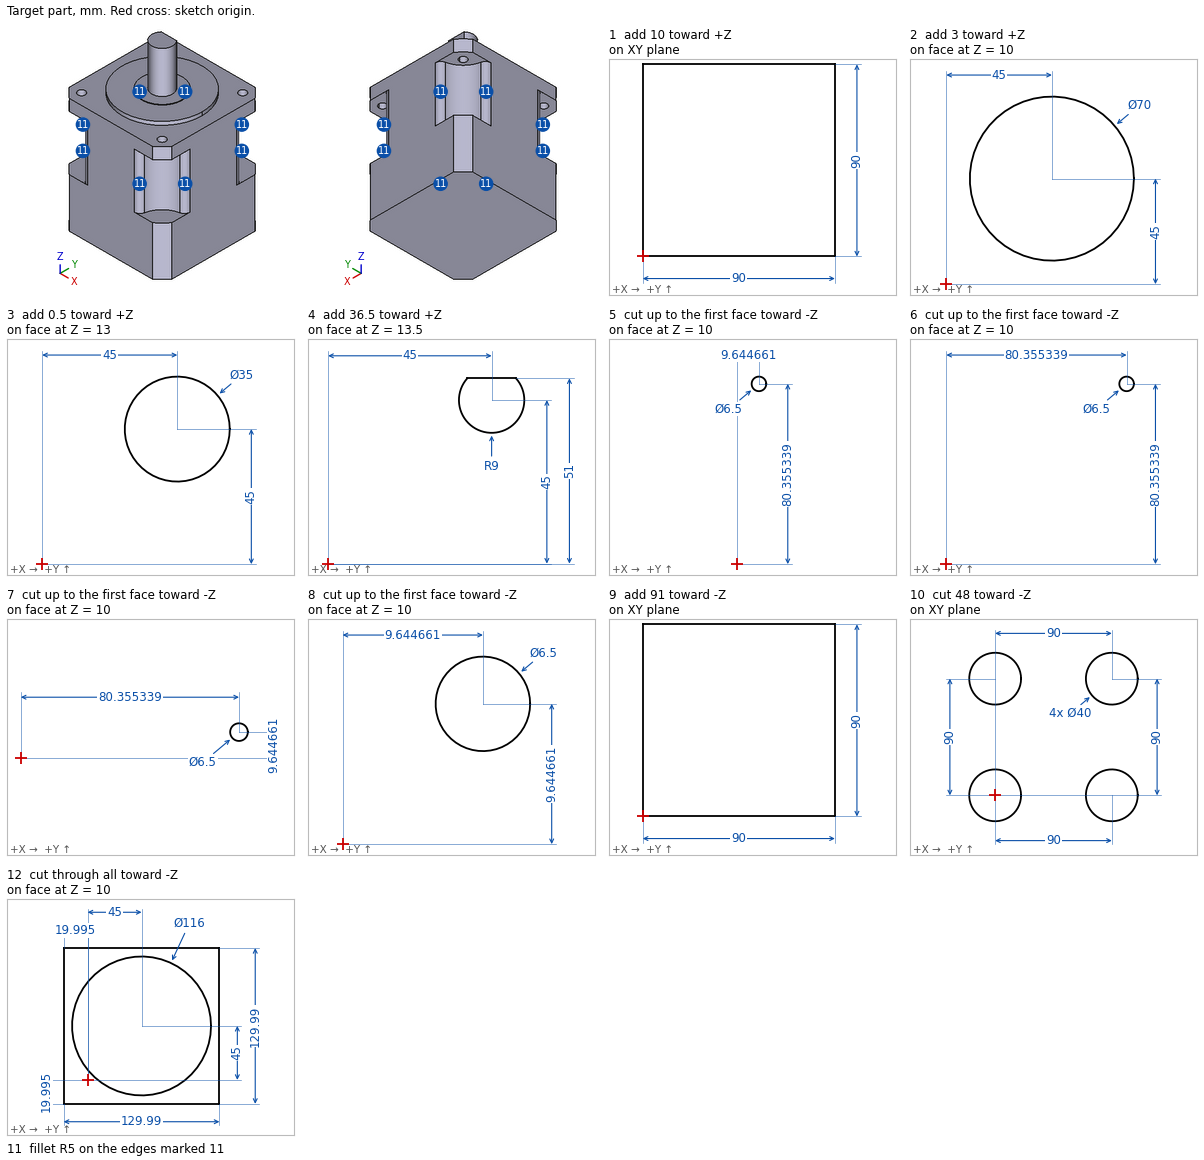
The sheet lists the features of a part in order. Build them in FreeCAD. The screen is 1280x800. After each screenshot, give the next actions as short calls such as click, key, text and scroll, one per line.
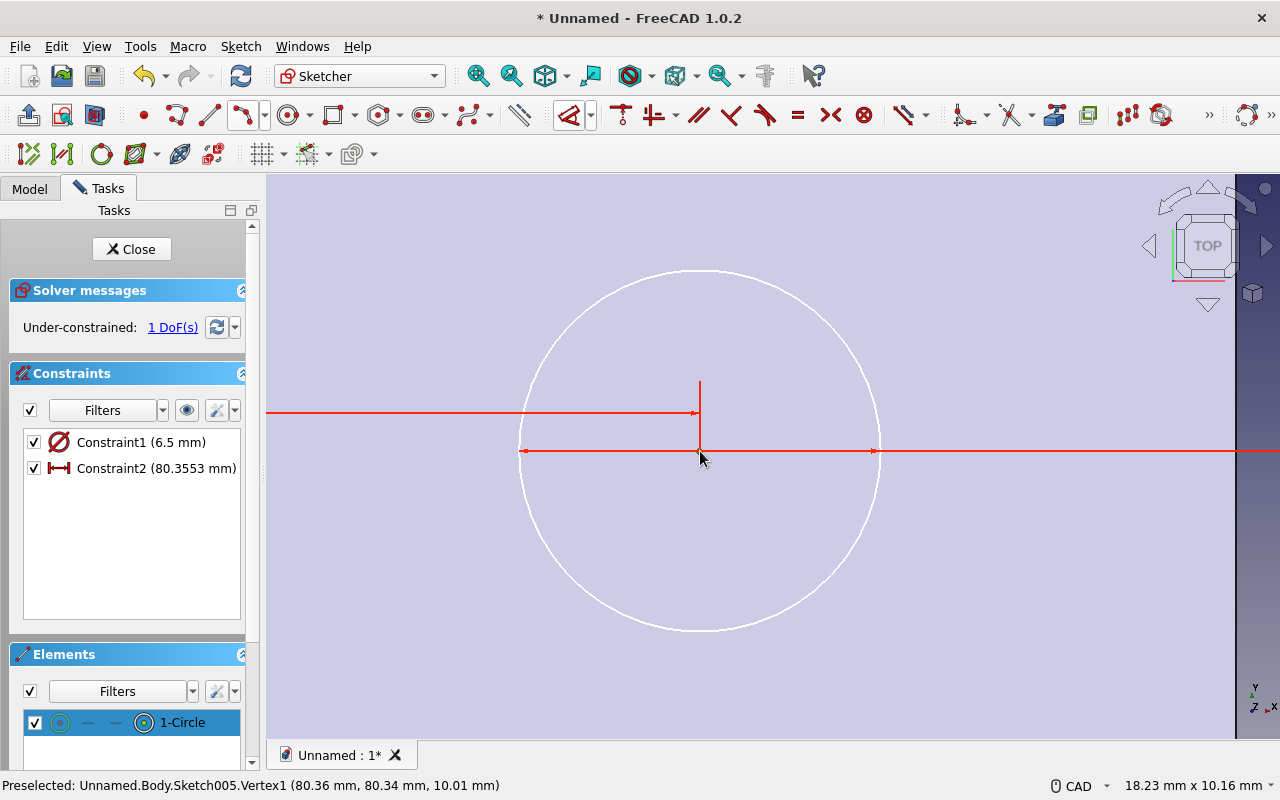
key(i)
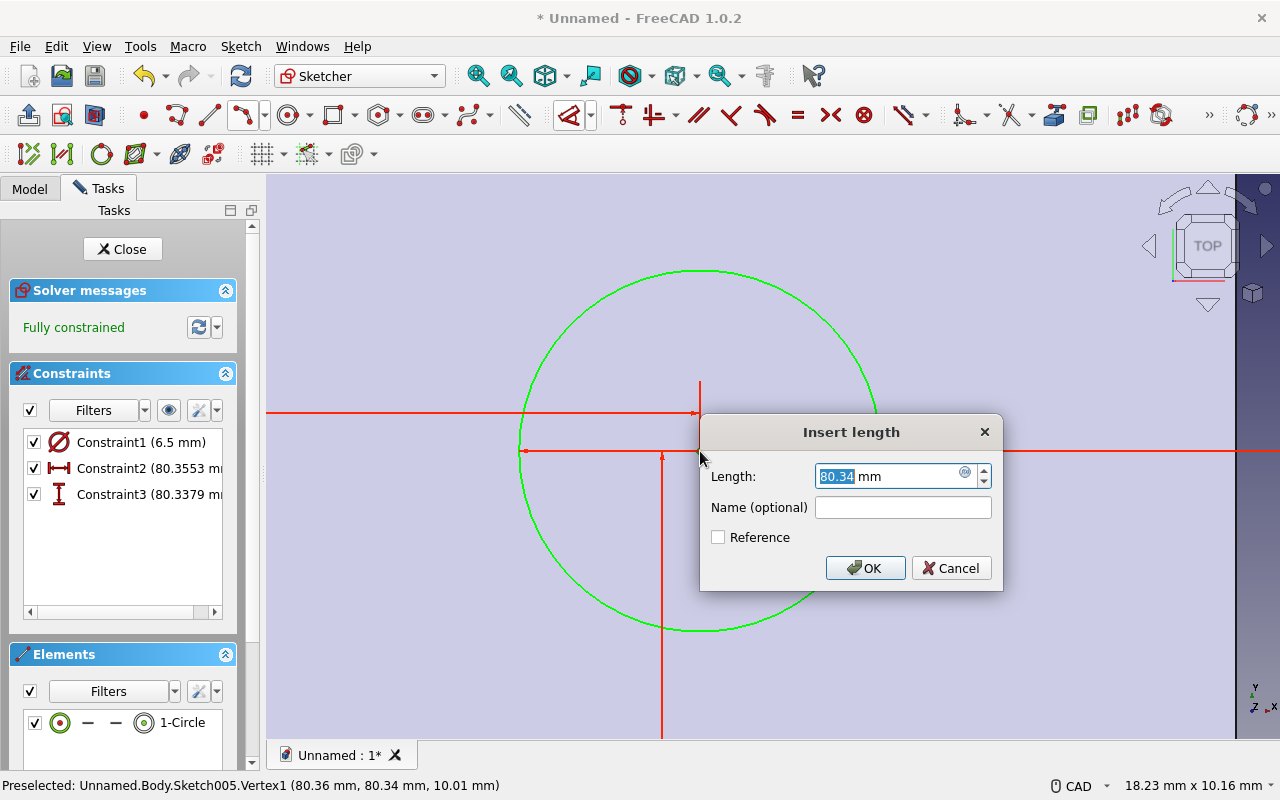
text(80.355339)
key(Return)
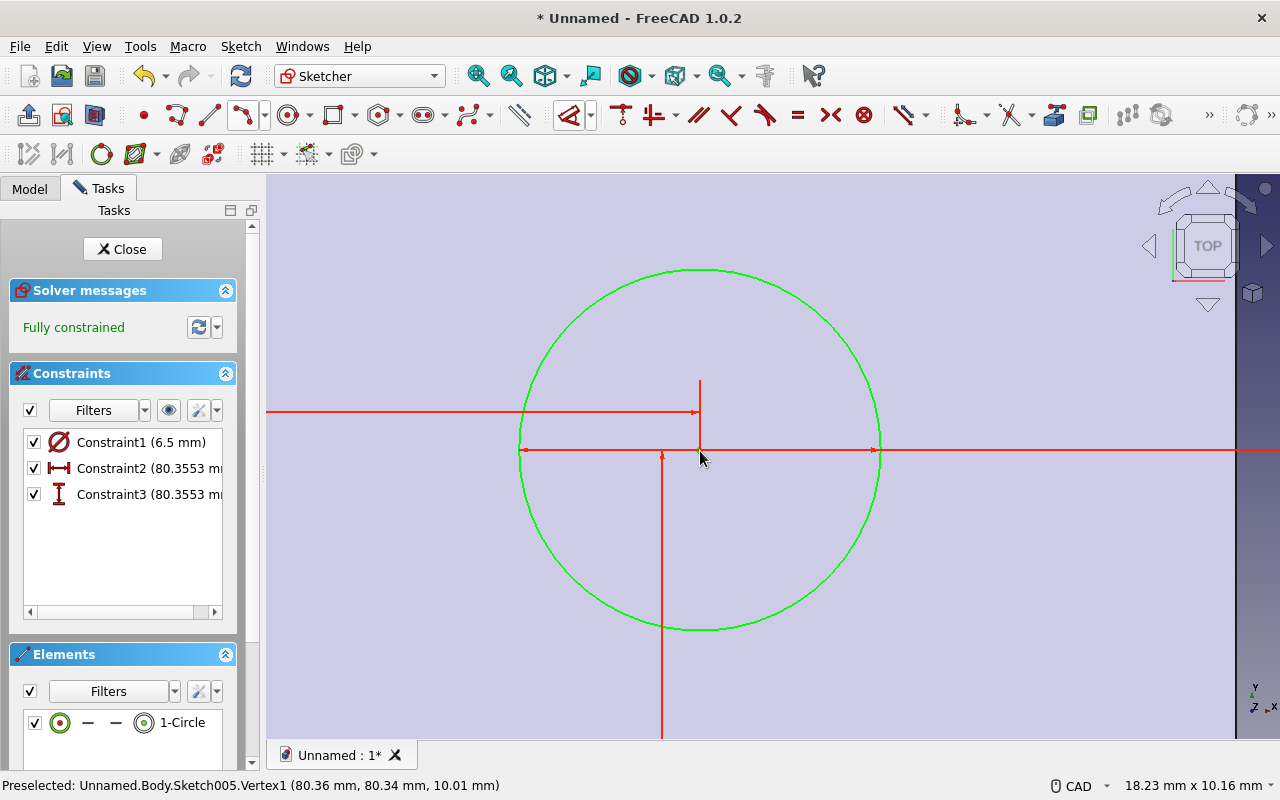
click(123, 249)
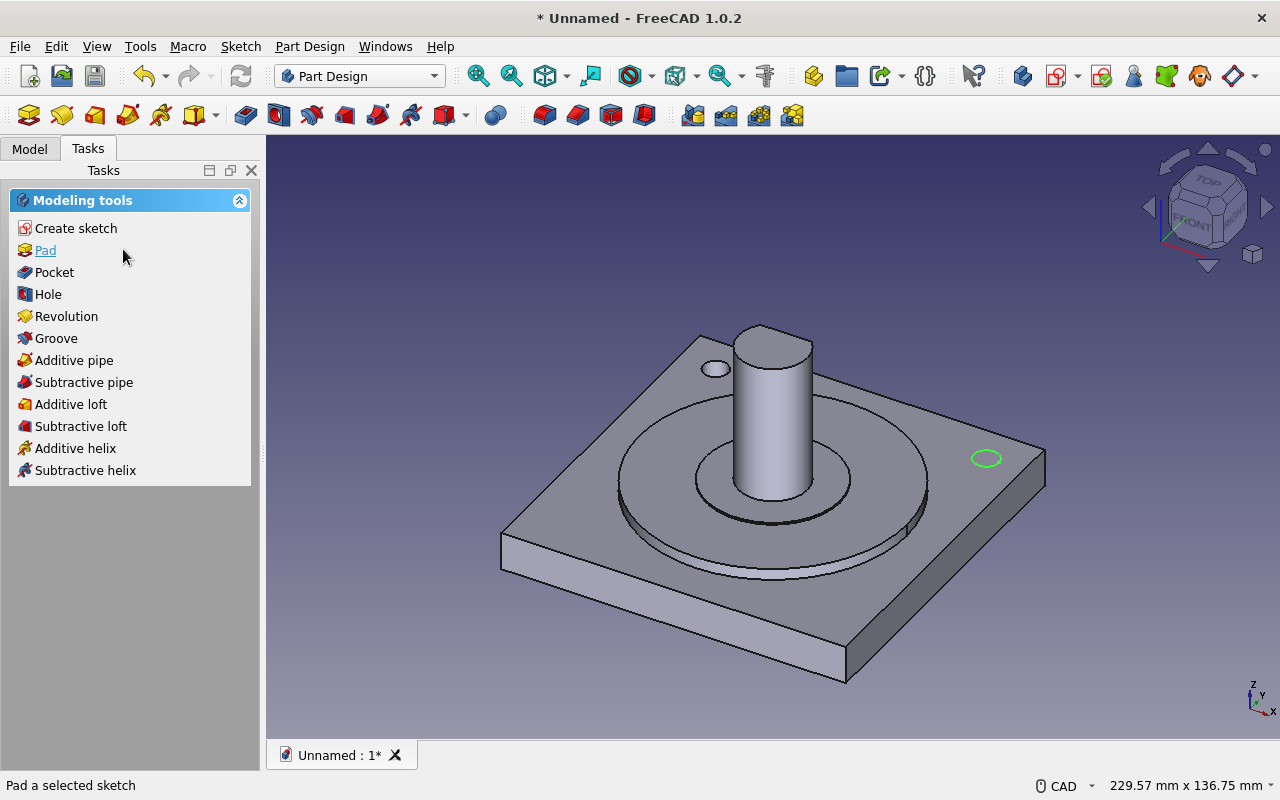
click(246, 116)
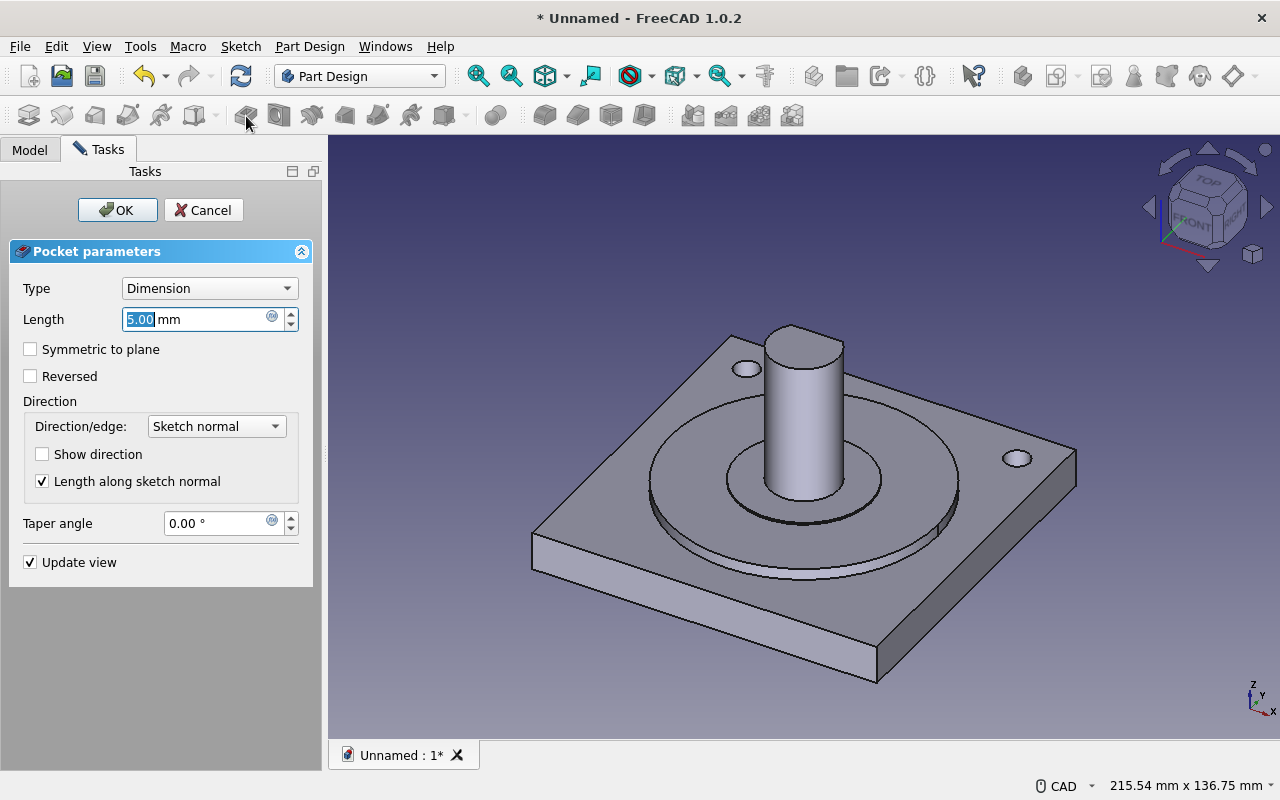
click(210, 288)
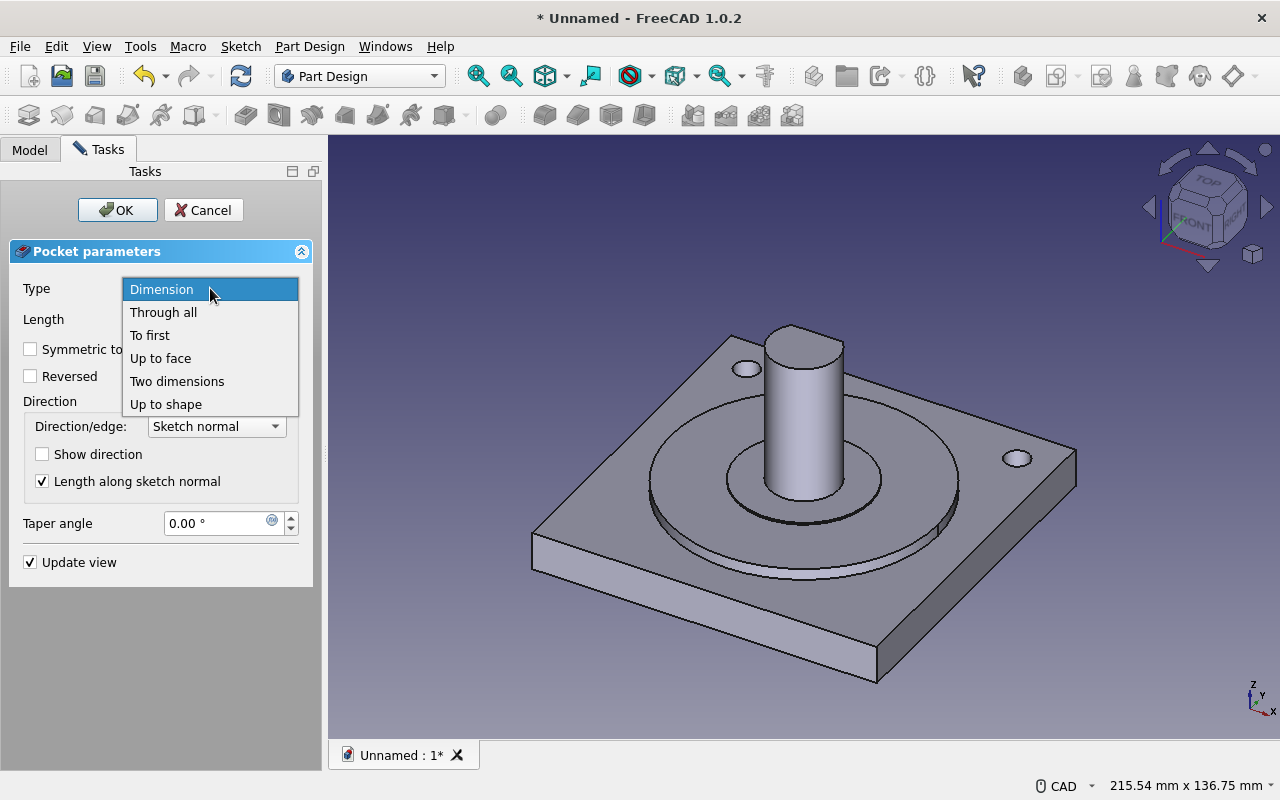
click(208, 336)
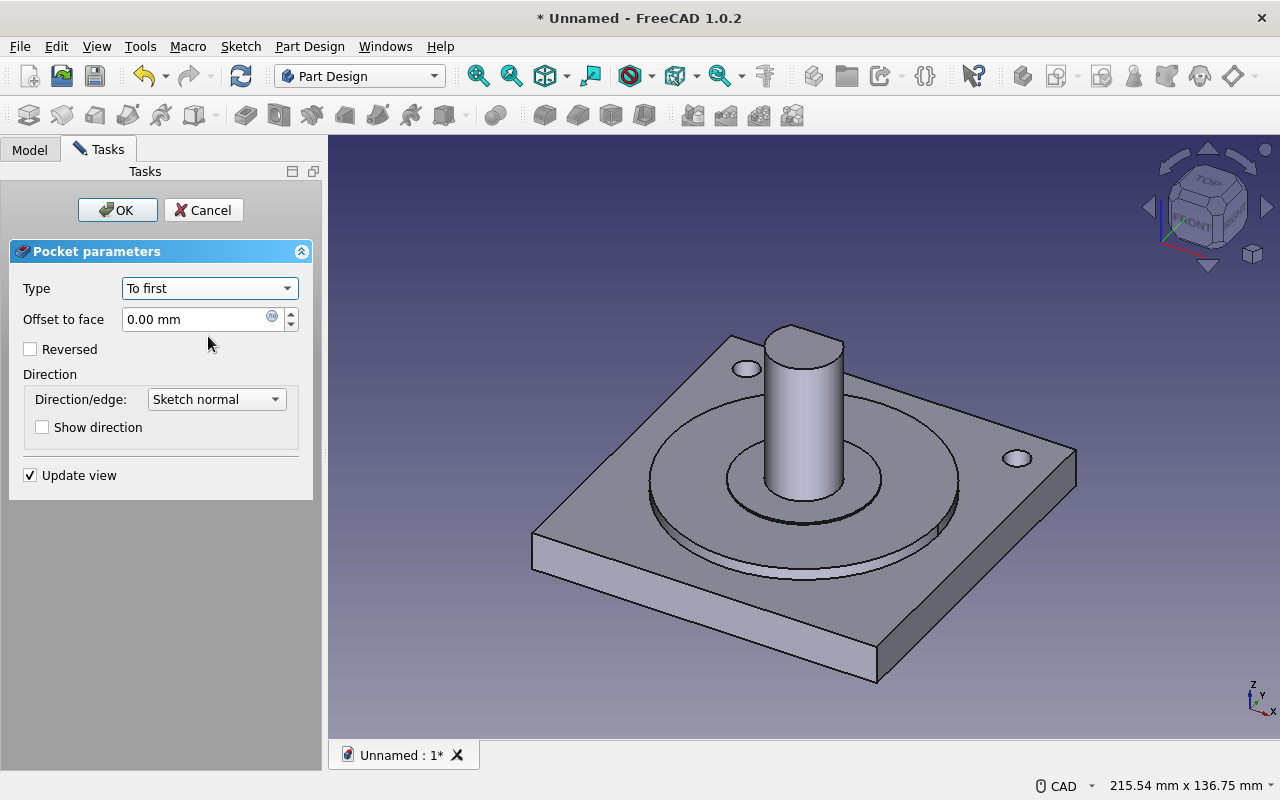
click(118, 210)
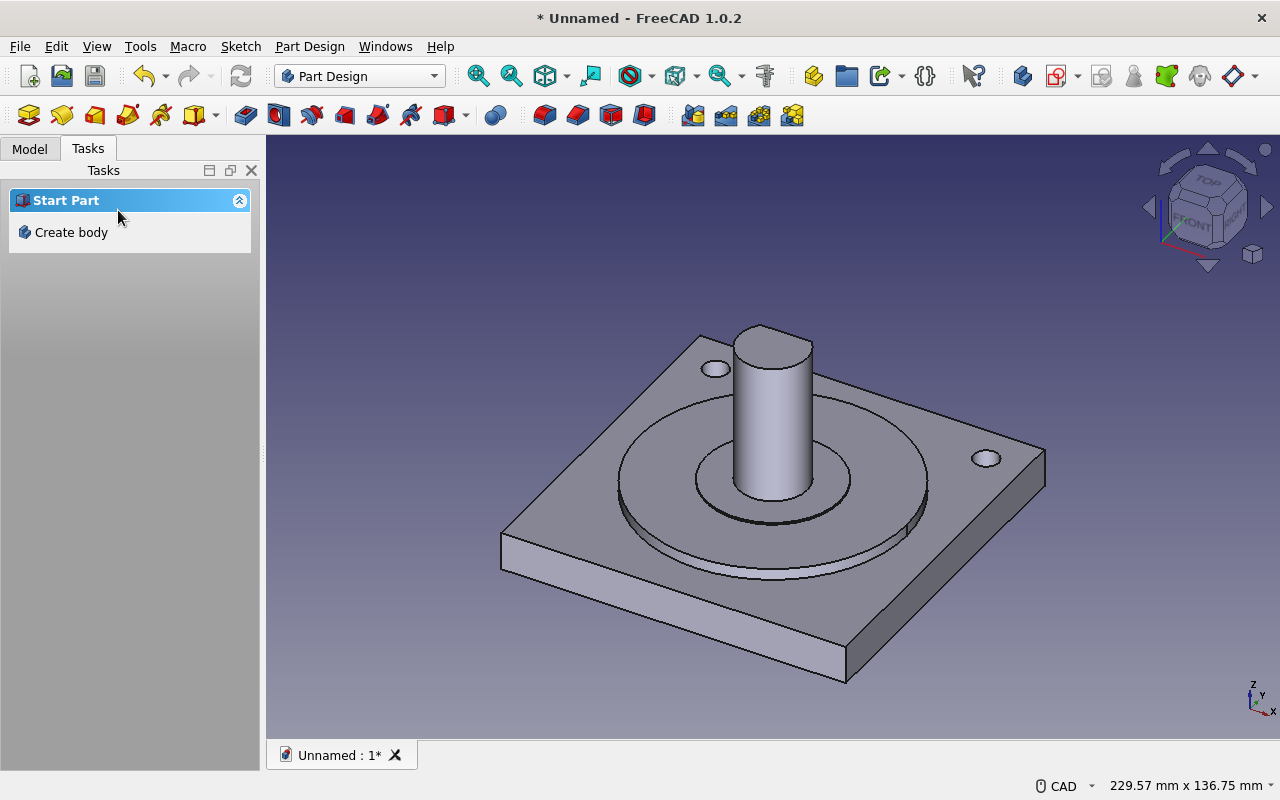
click(977, 483)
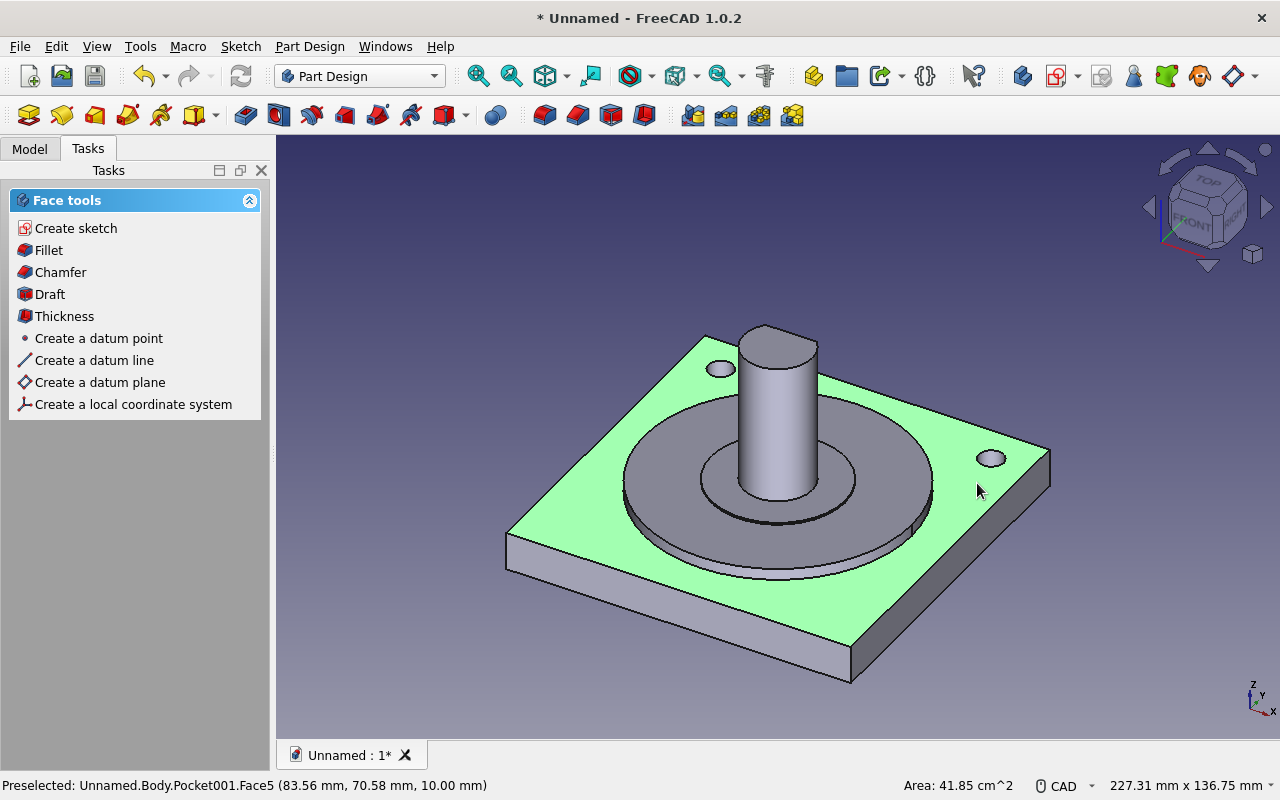
click(1056, 76)